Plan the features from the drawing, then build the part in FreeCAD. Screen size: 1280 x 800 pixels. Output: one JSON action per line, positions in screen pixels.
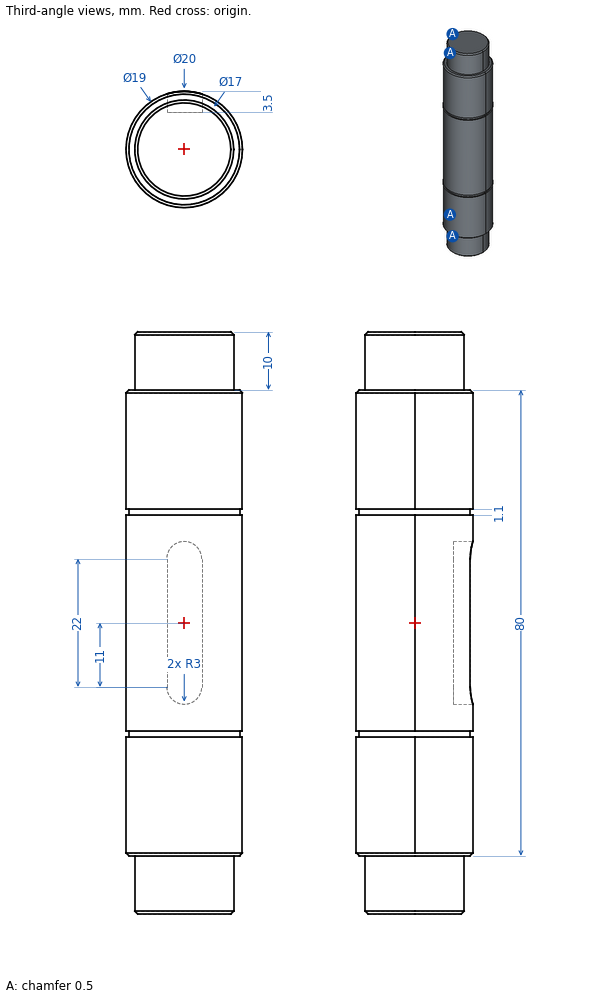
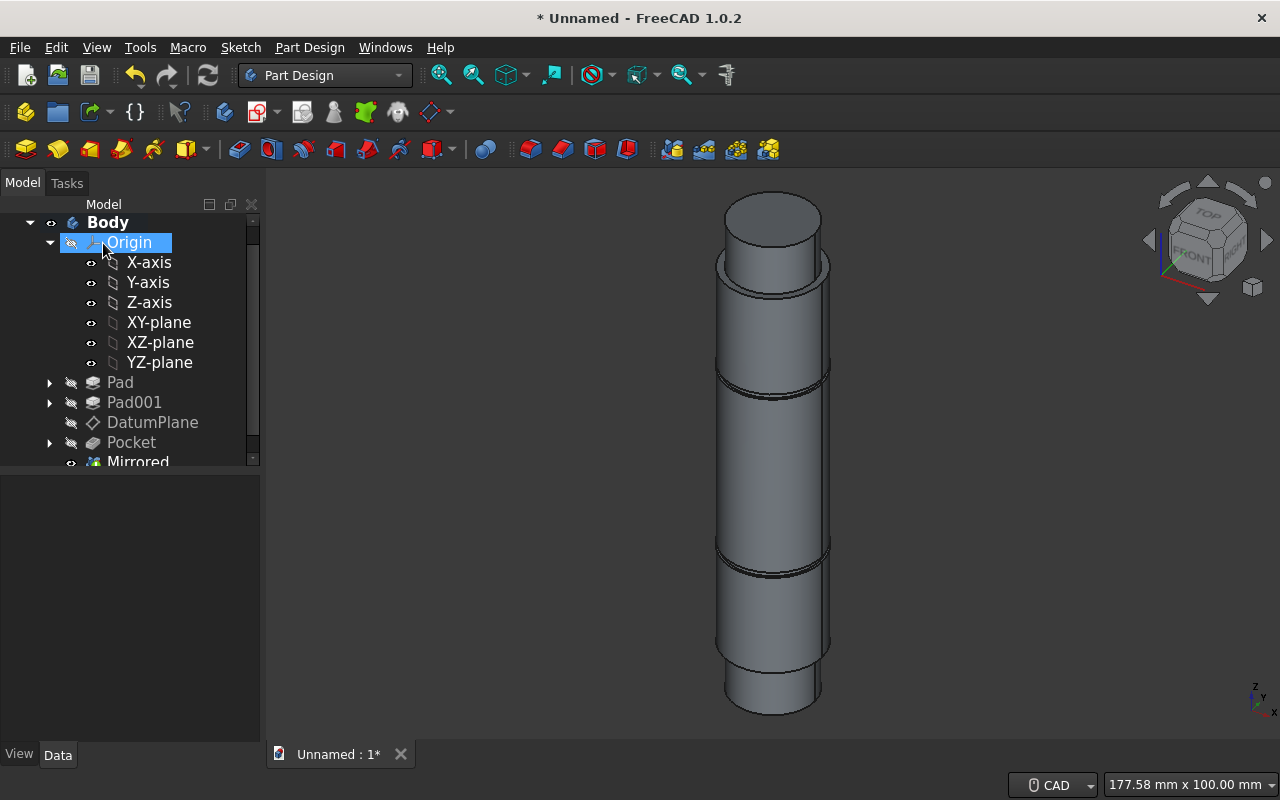
{"action": "left_click", "coordinate": [716, 269]}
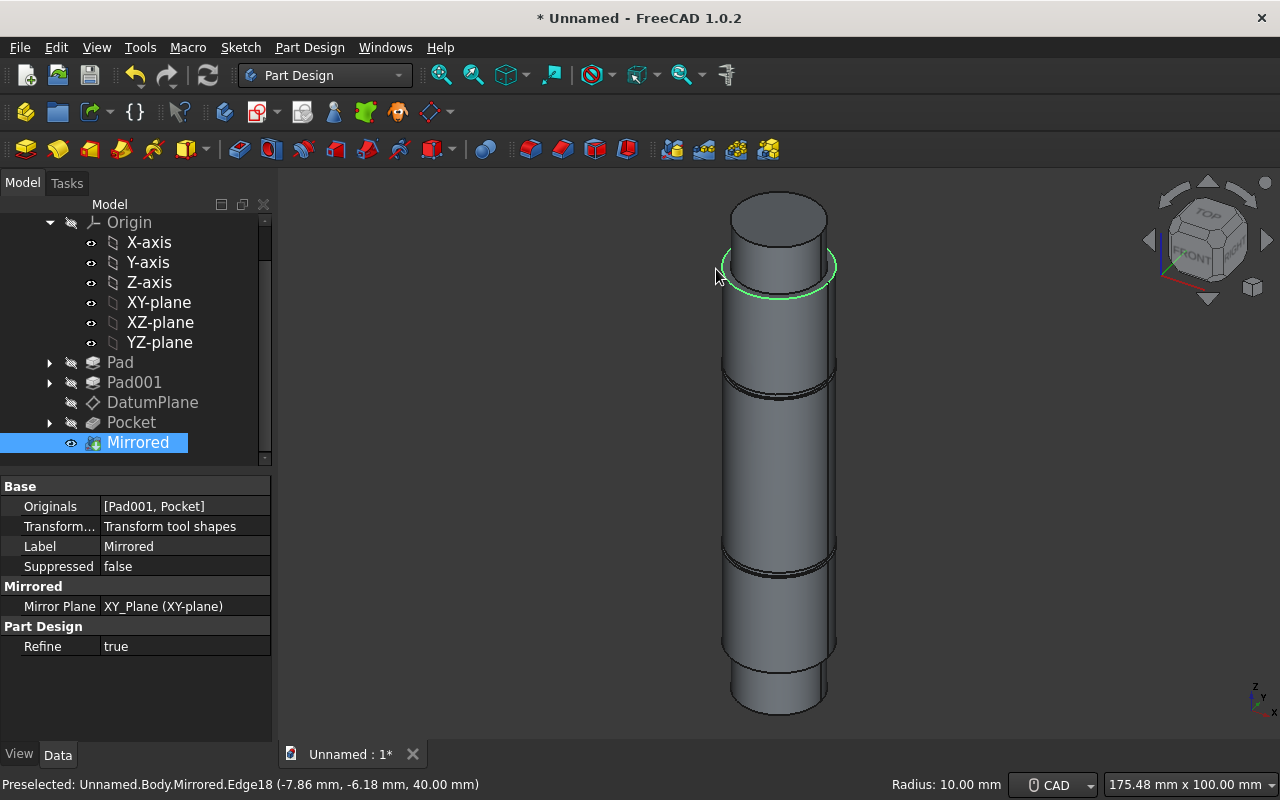
{"action": "left_click", "coordinate": [731, 222], "text": "ctrl"}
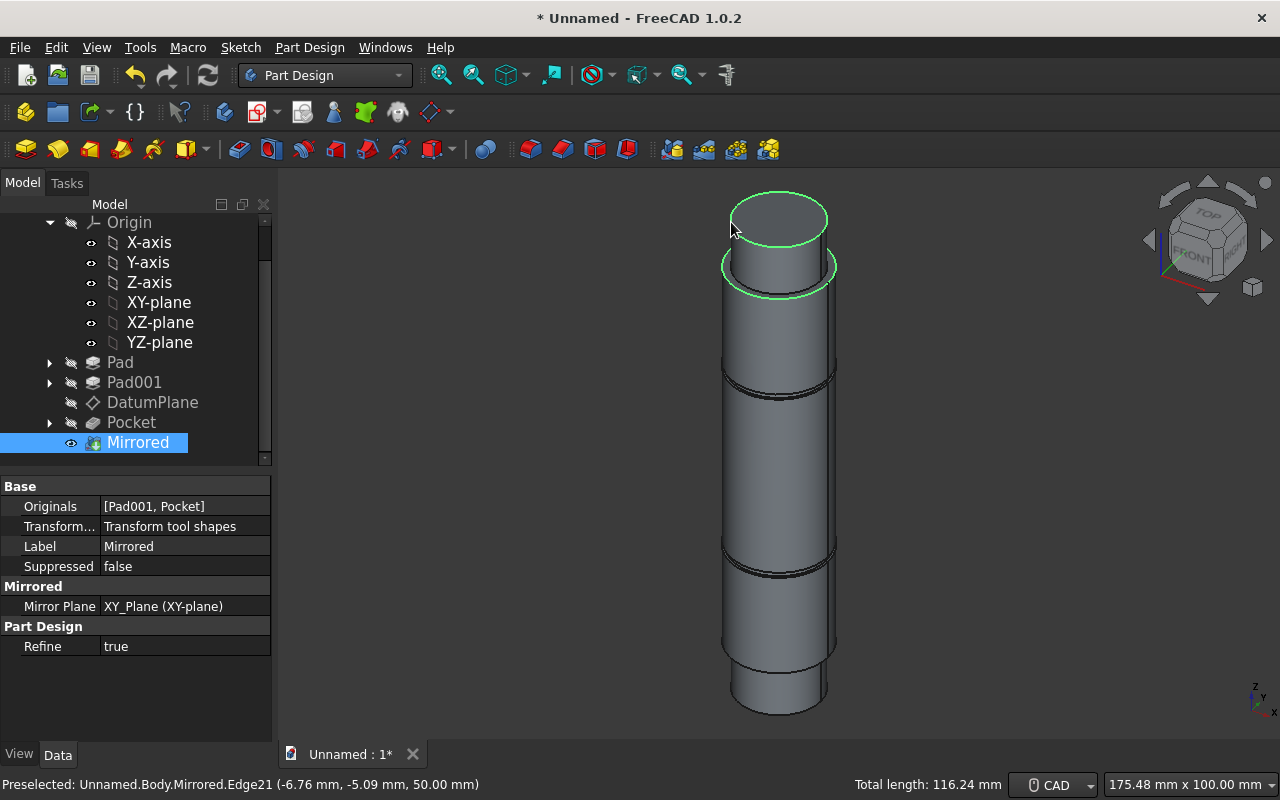
{"action": "key", "text": "0"}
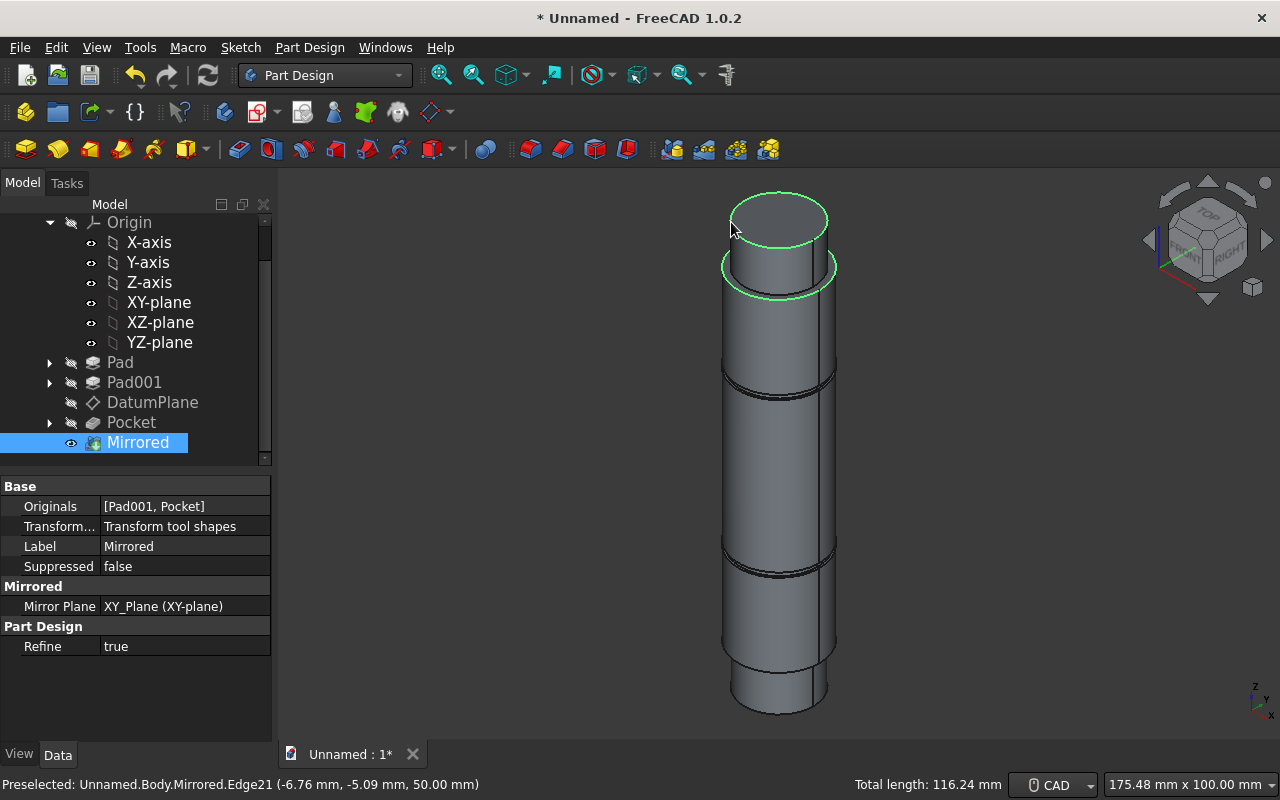
{"action": "key", "text": "2"}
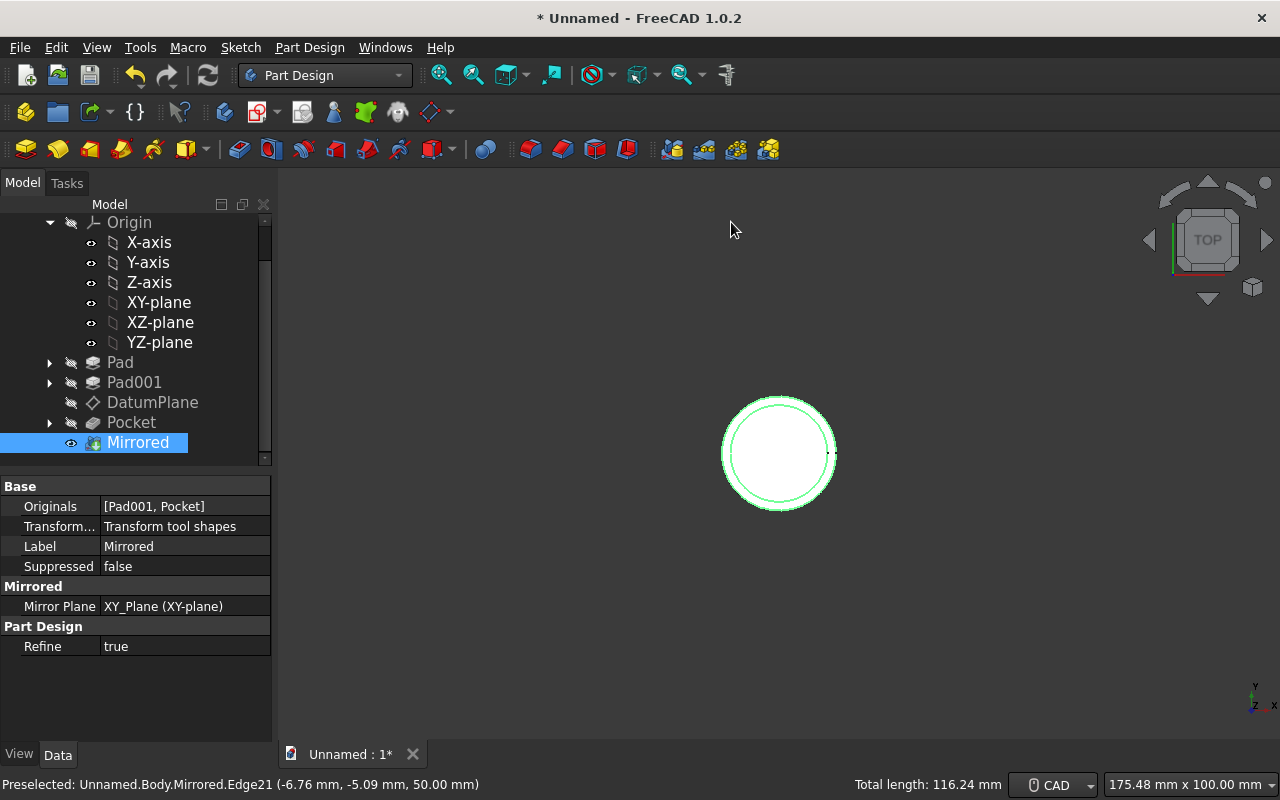
{"action": "key", "text": "v f"}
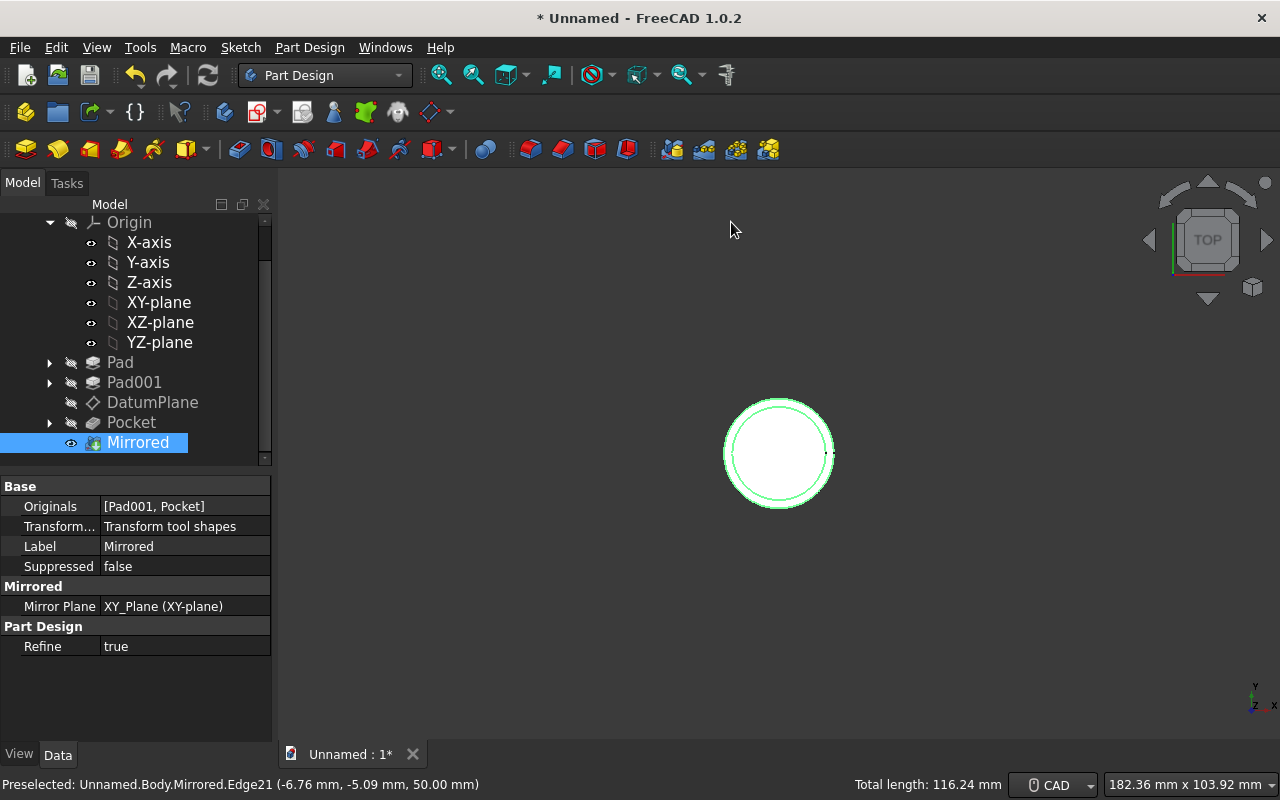
{"action": "key", "text": "1"}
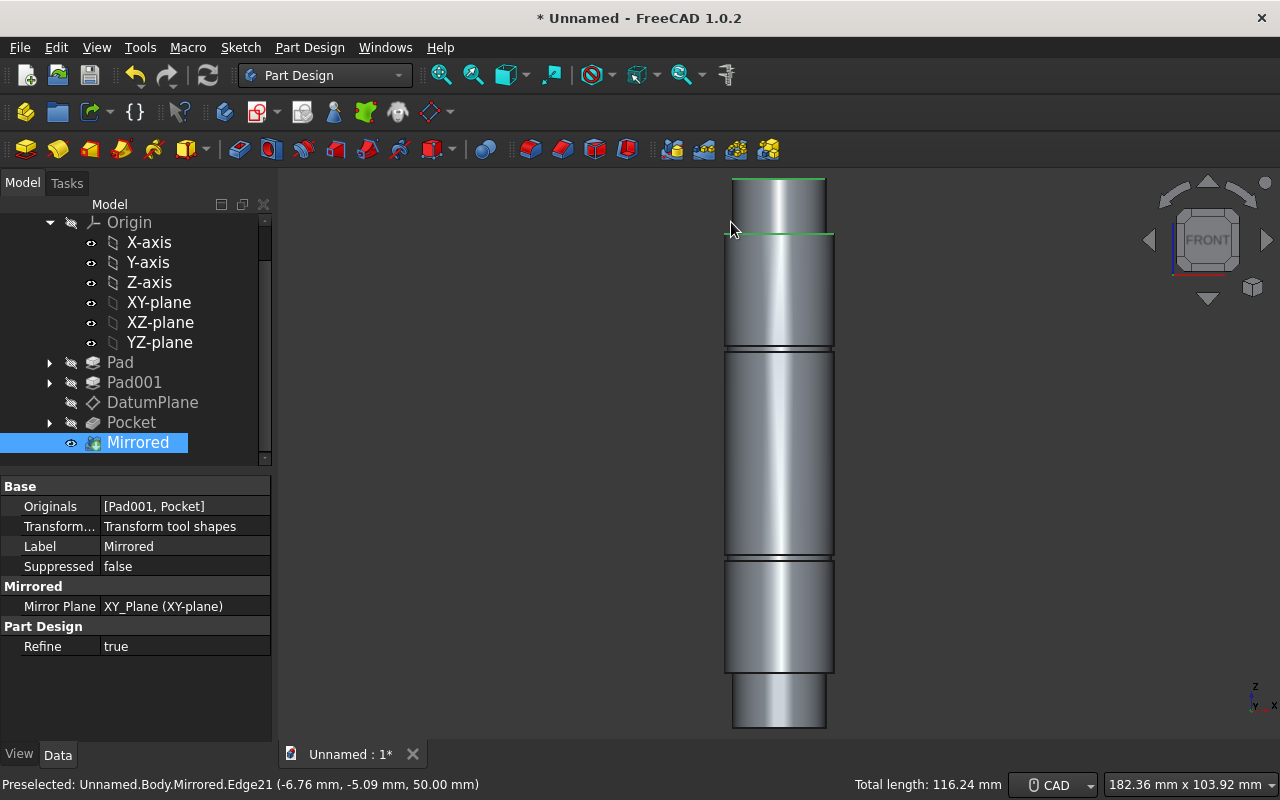
{"action": "left_click", "coordinate": [735, 672], "text": "ctrl"}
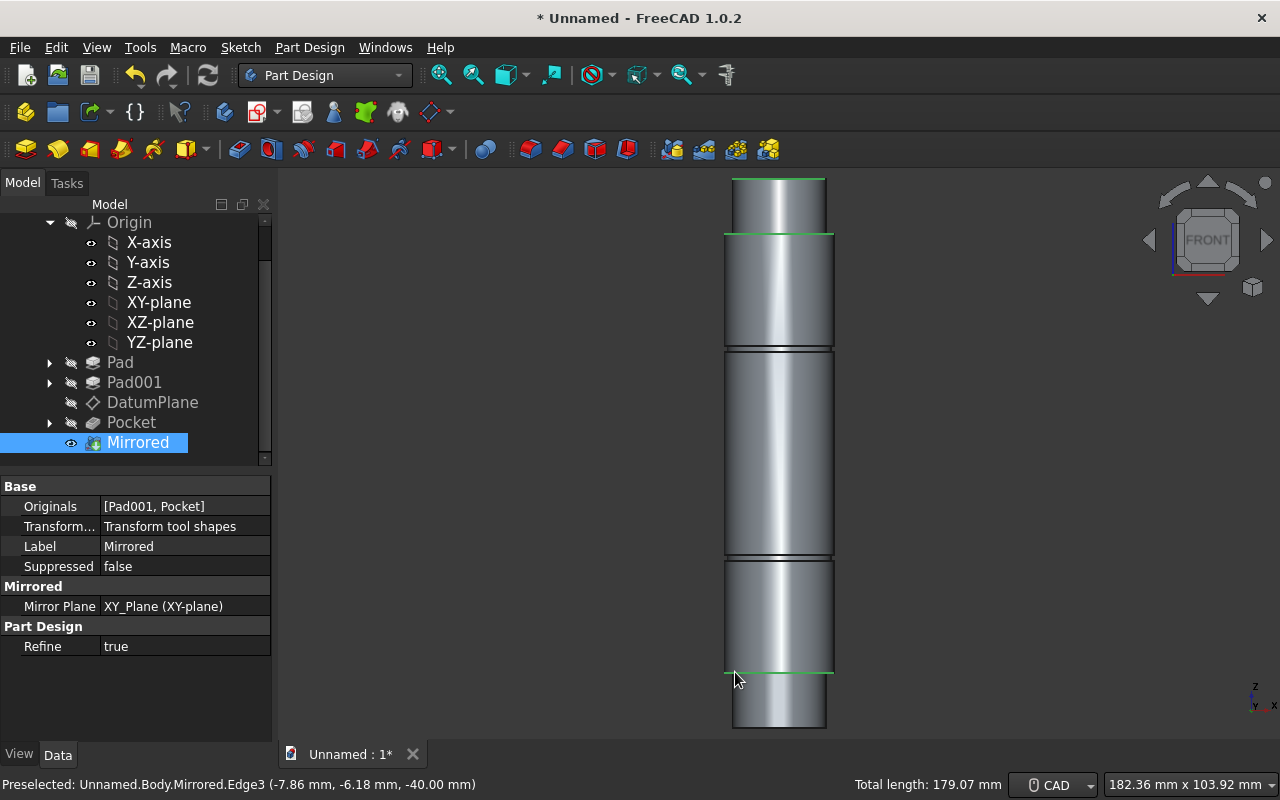
{"action": "key", "text": "3"}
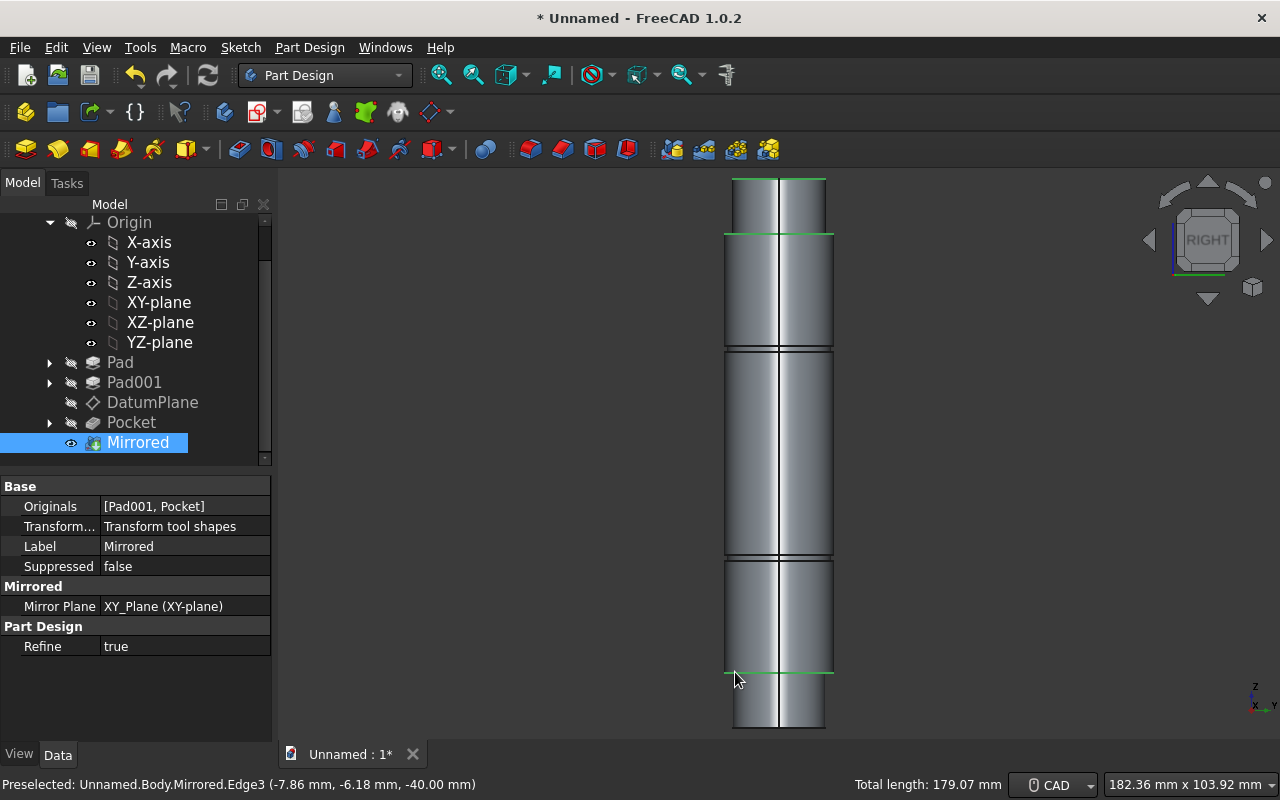
{"action": "key", "text": "5"}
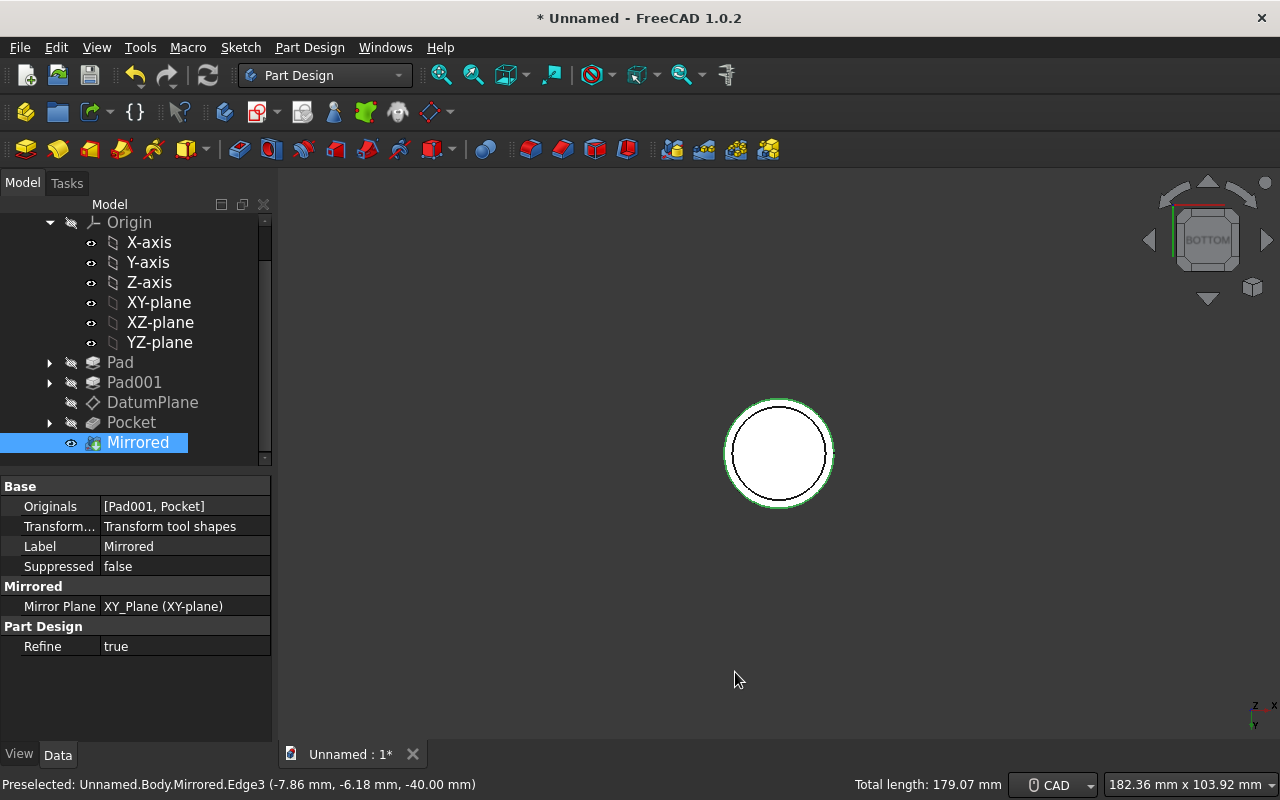
{"action": "left_click", "coordinate": [442, 76]}